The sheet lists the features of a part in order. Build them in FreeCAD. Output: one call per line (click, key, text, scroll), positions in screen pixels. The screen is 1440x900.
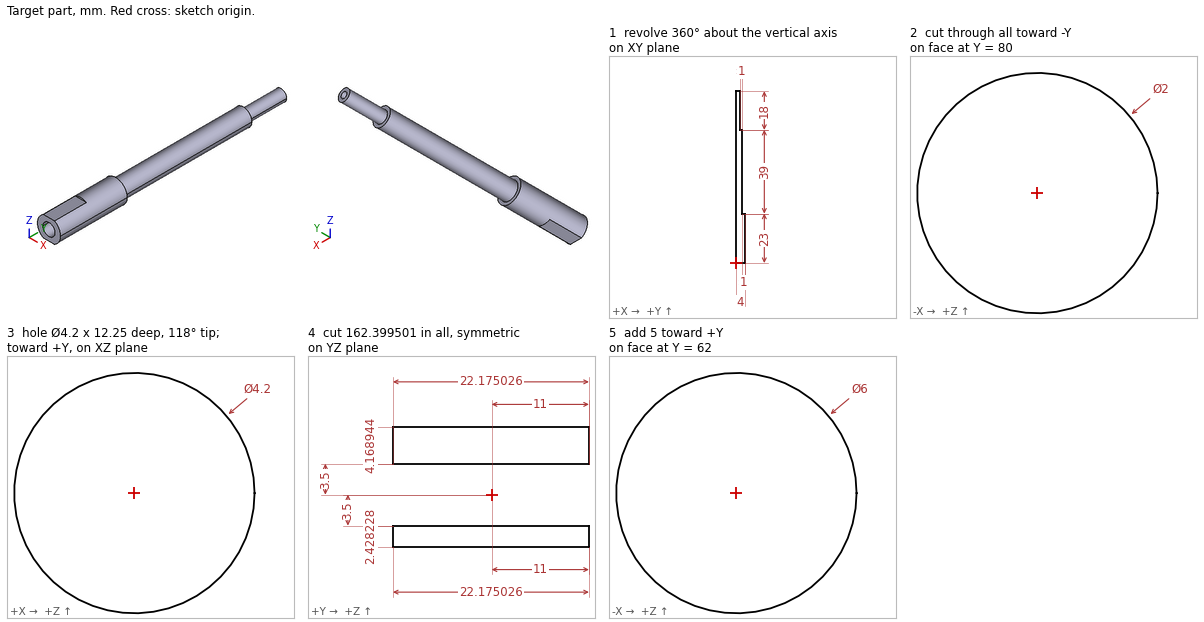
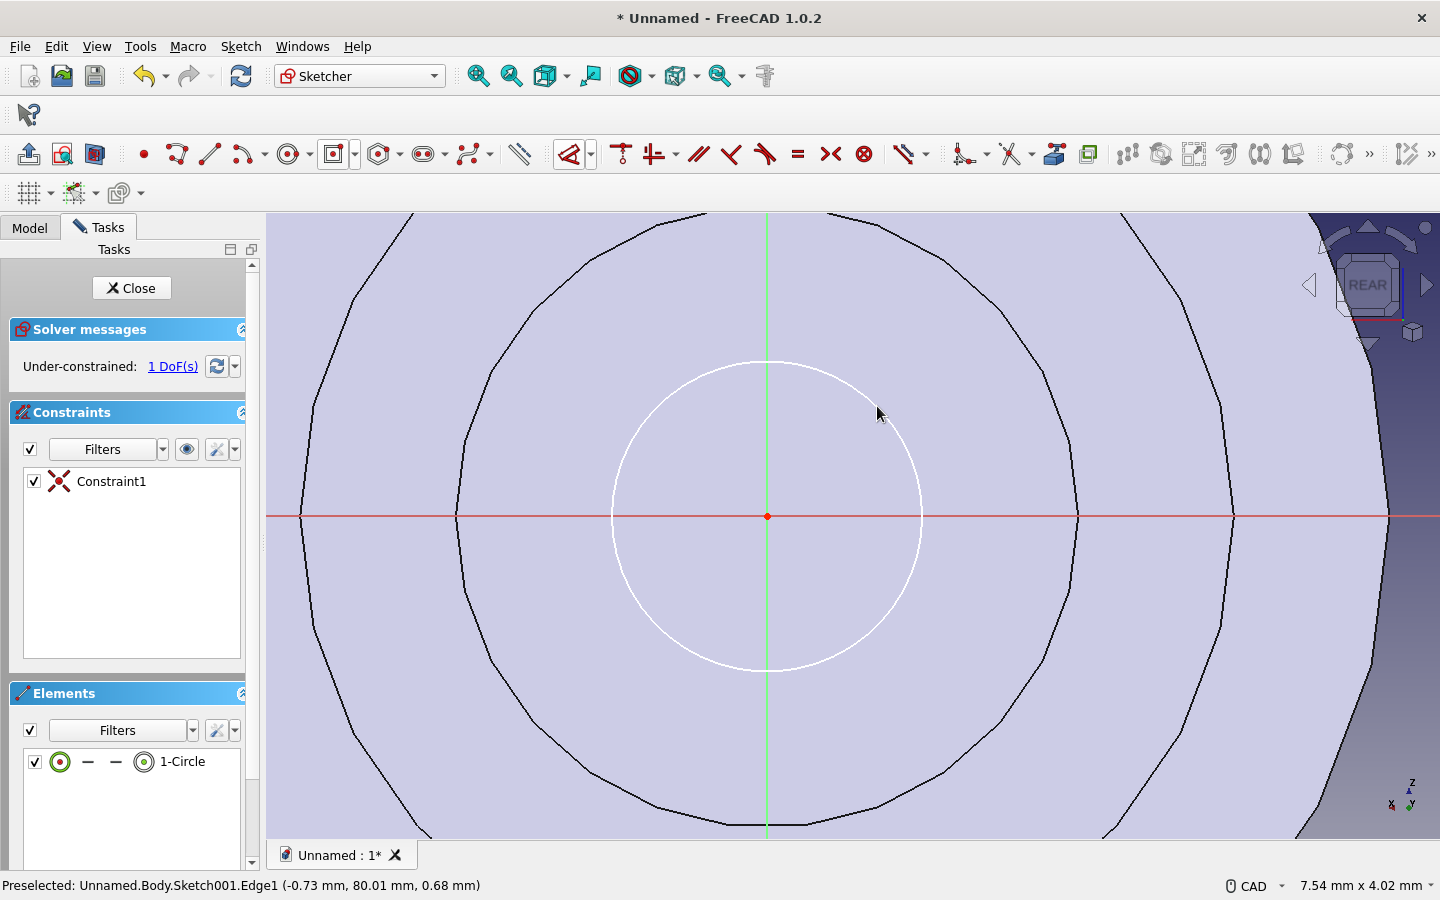
click(876, 406)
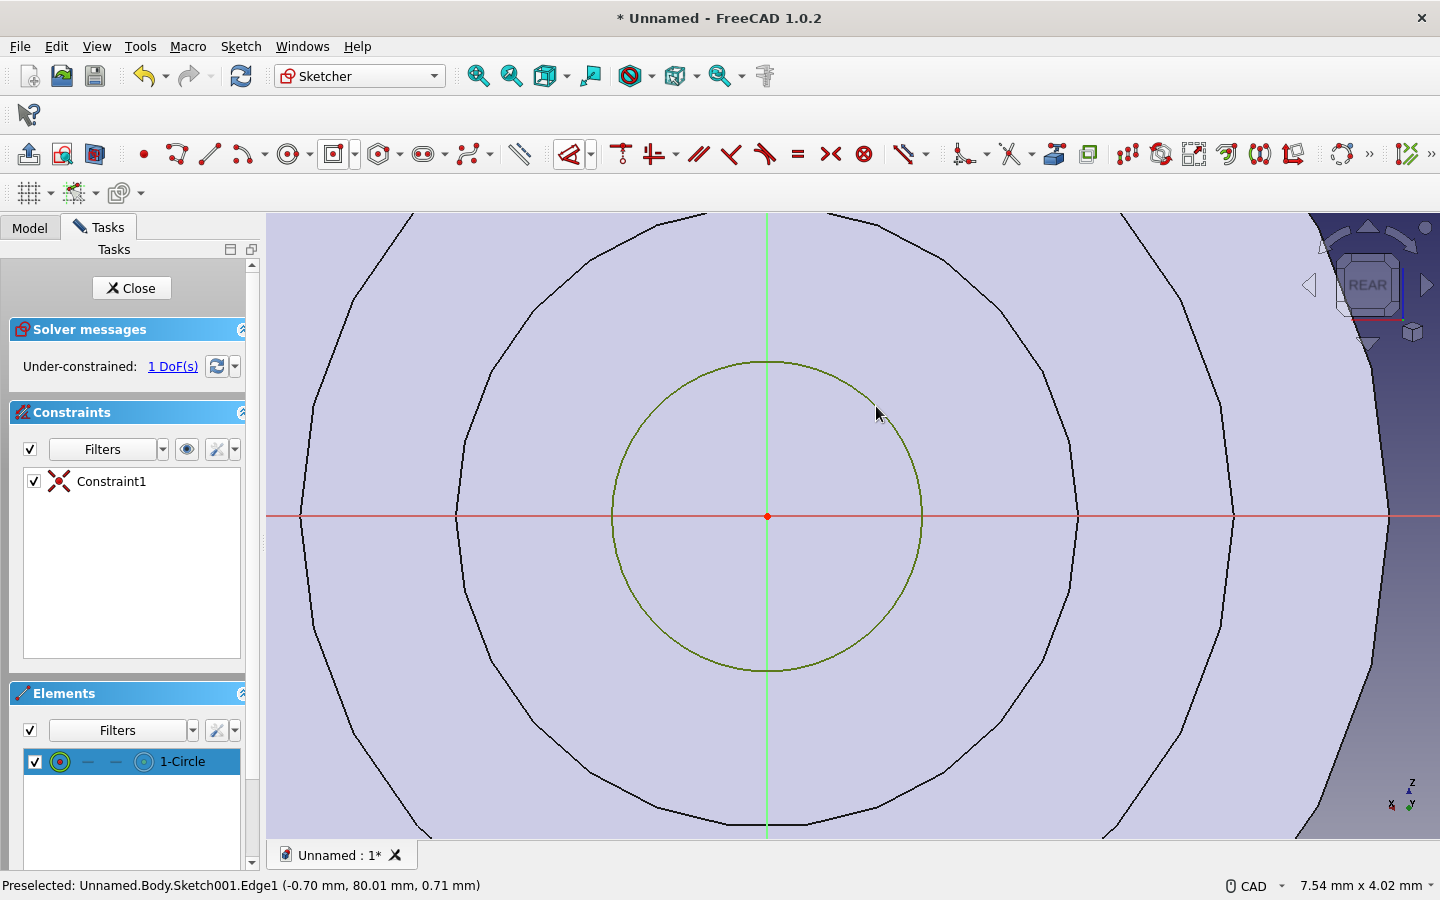
key(k)
key(o)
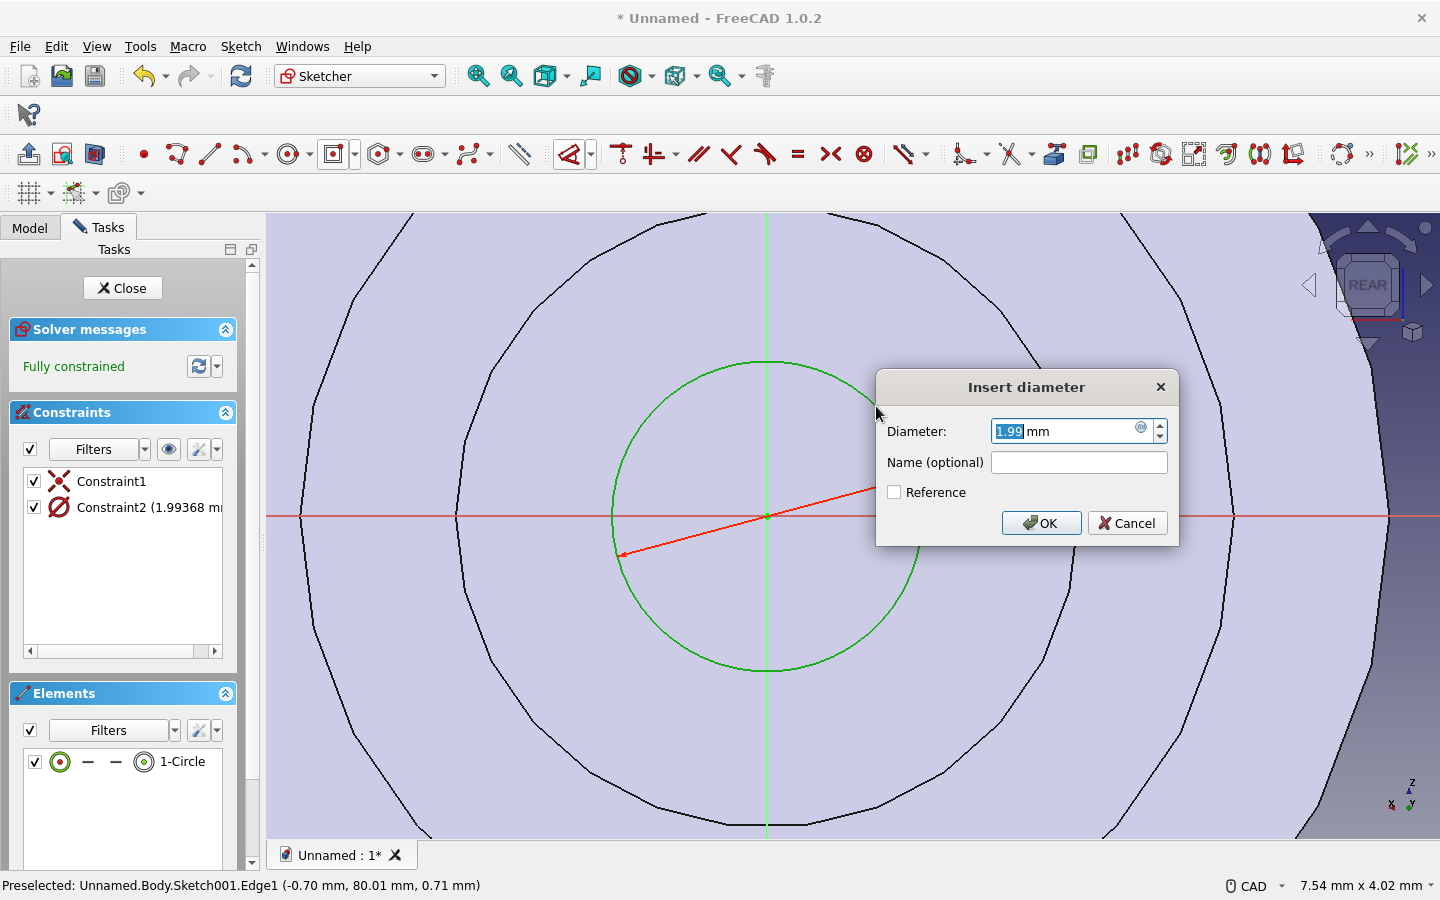
text(2)
key(Return)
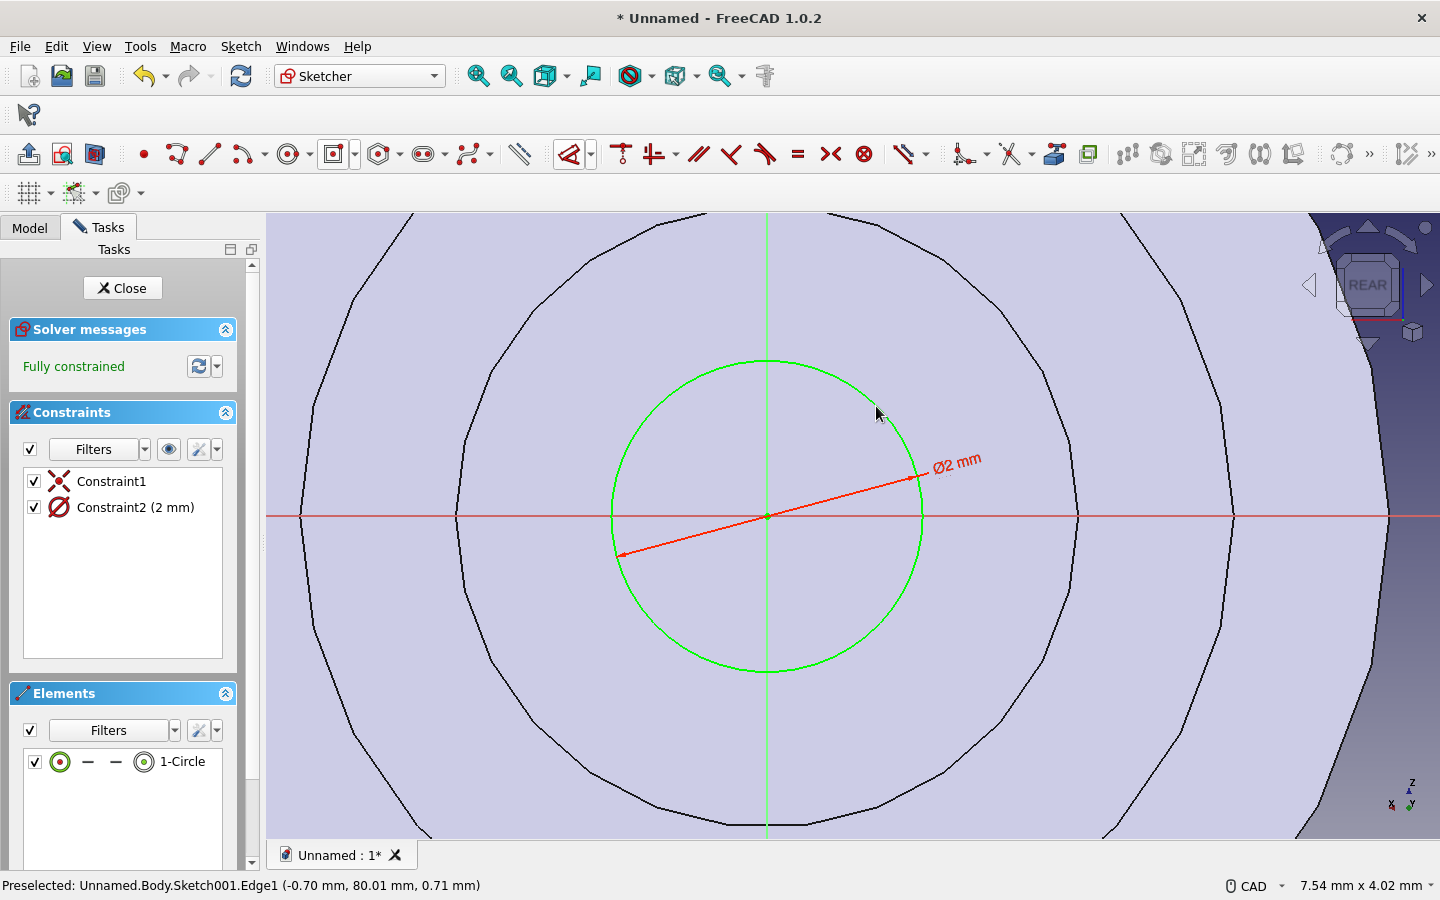
click(123, 288)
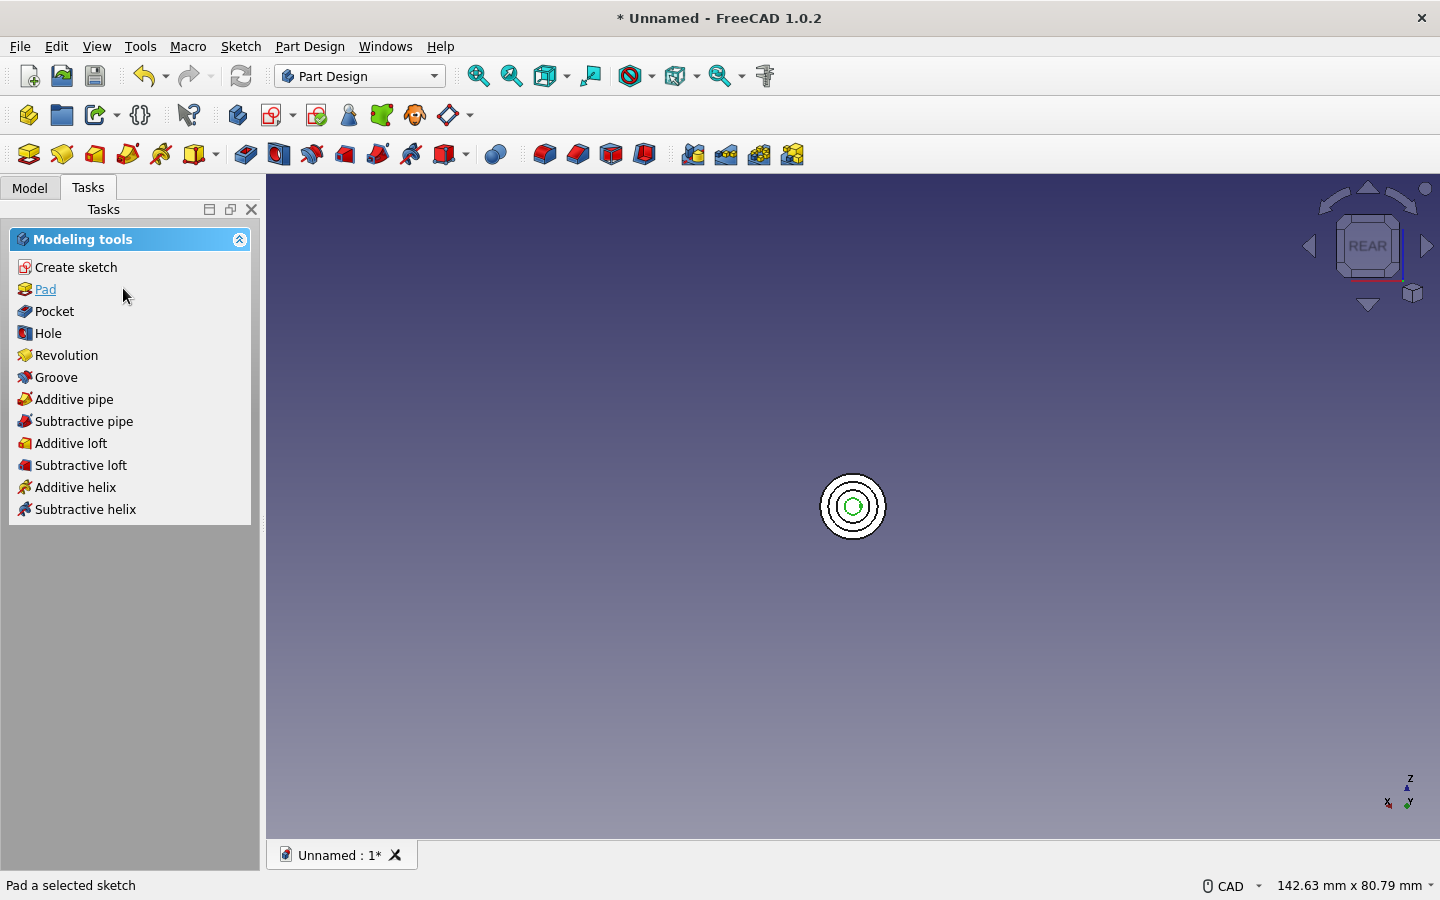
click(246, 154)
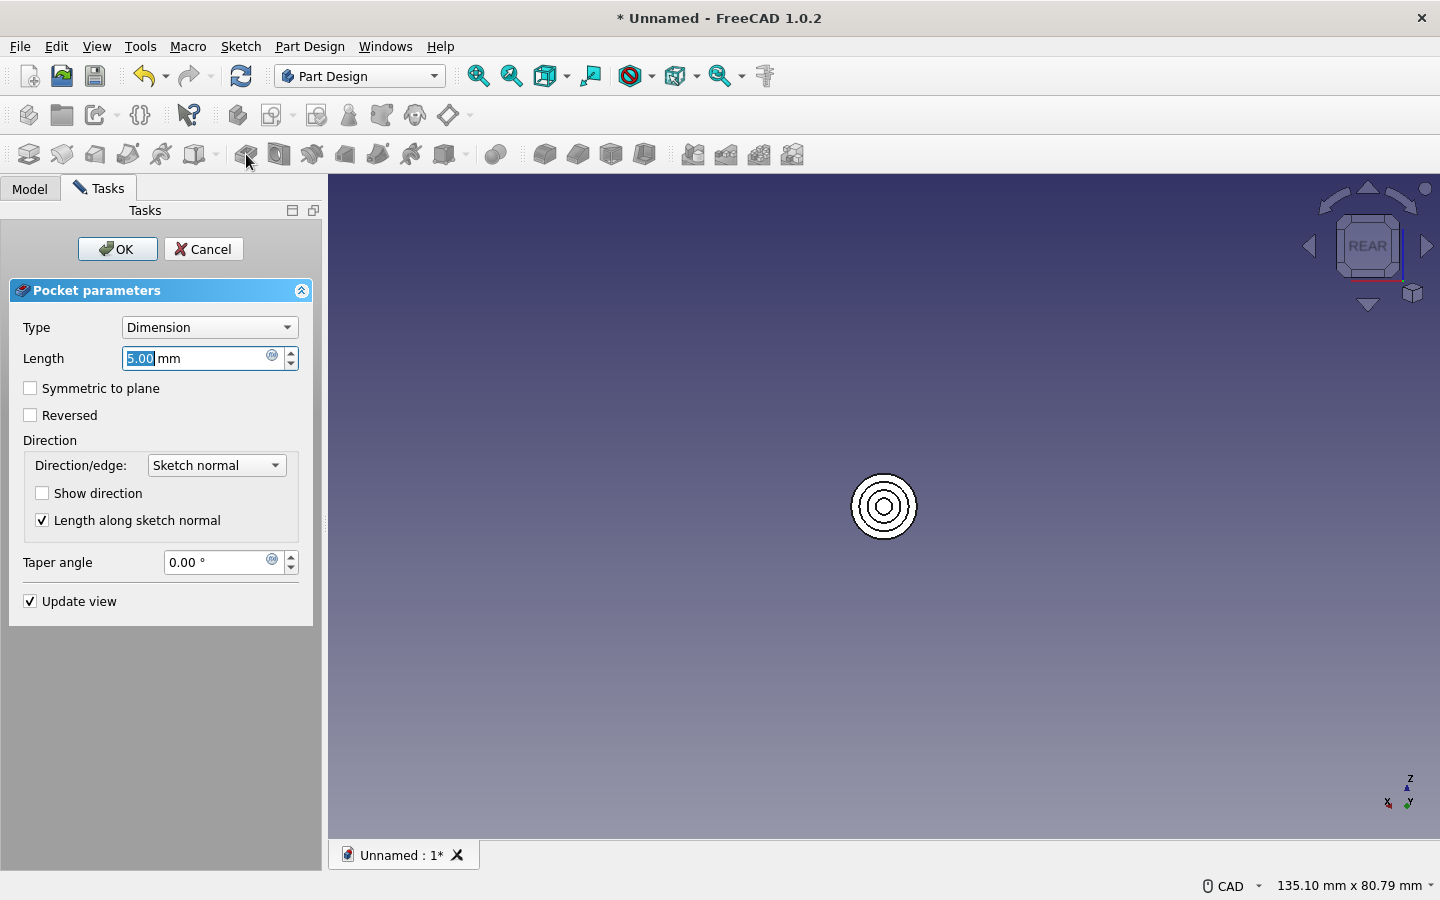
click(210, 328)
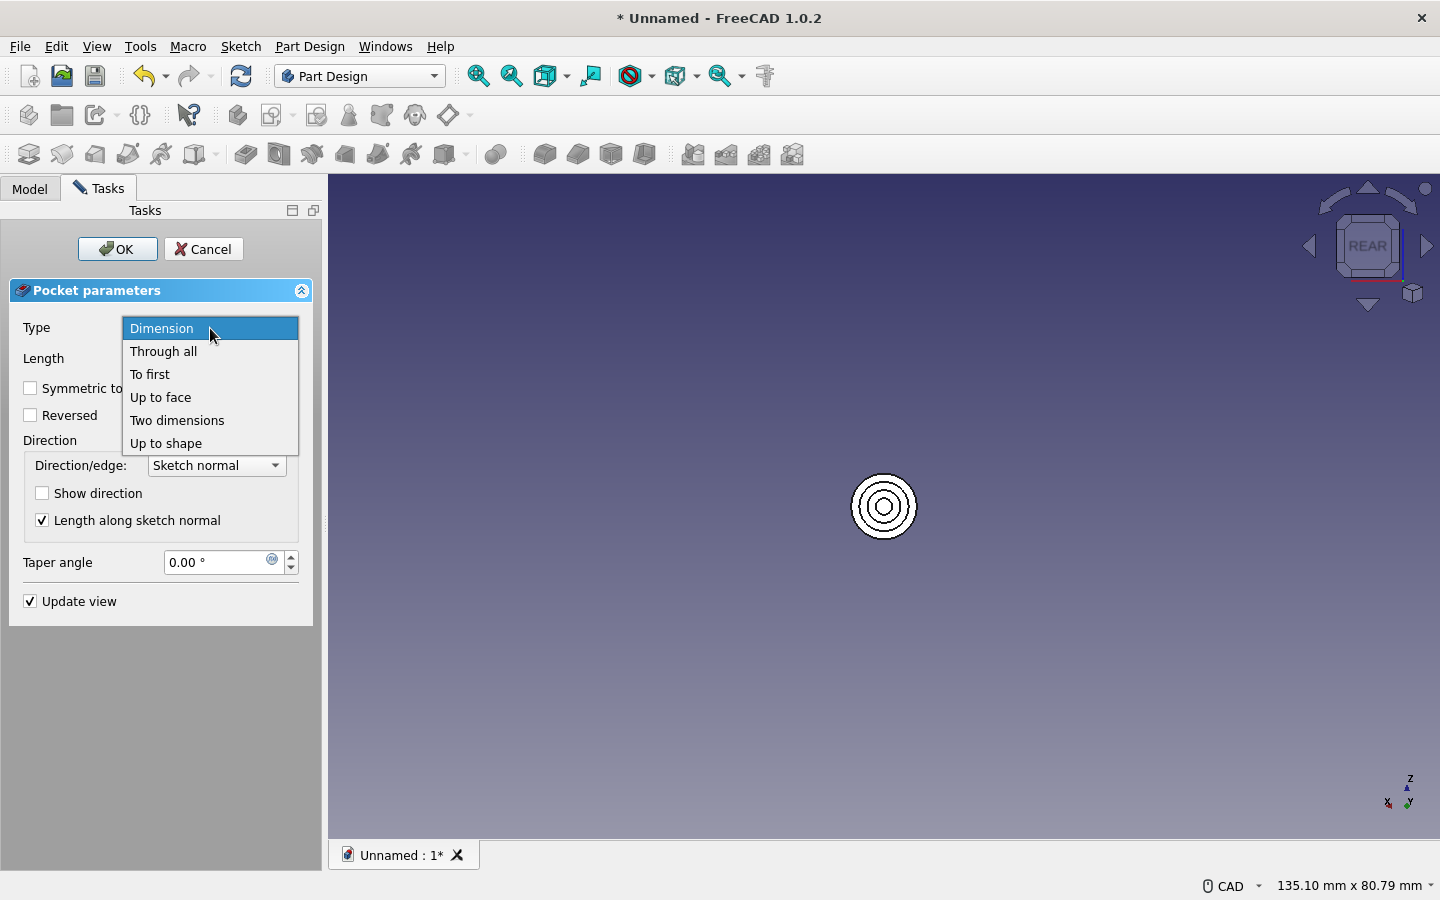
click(208, 352)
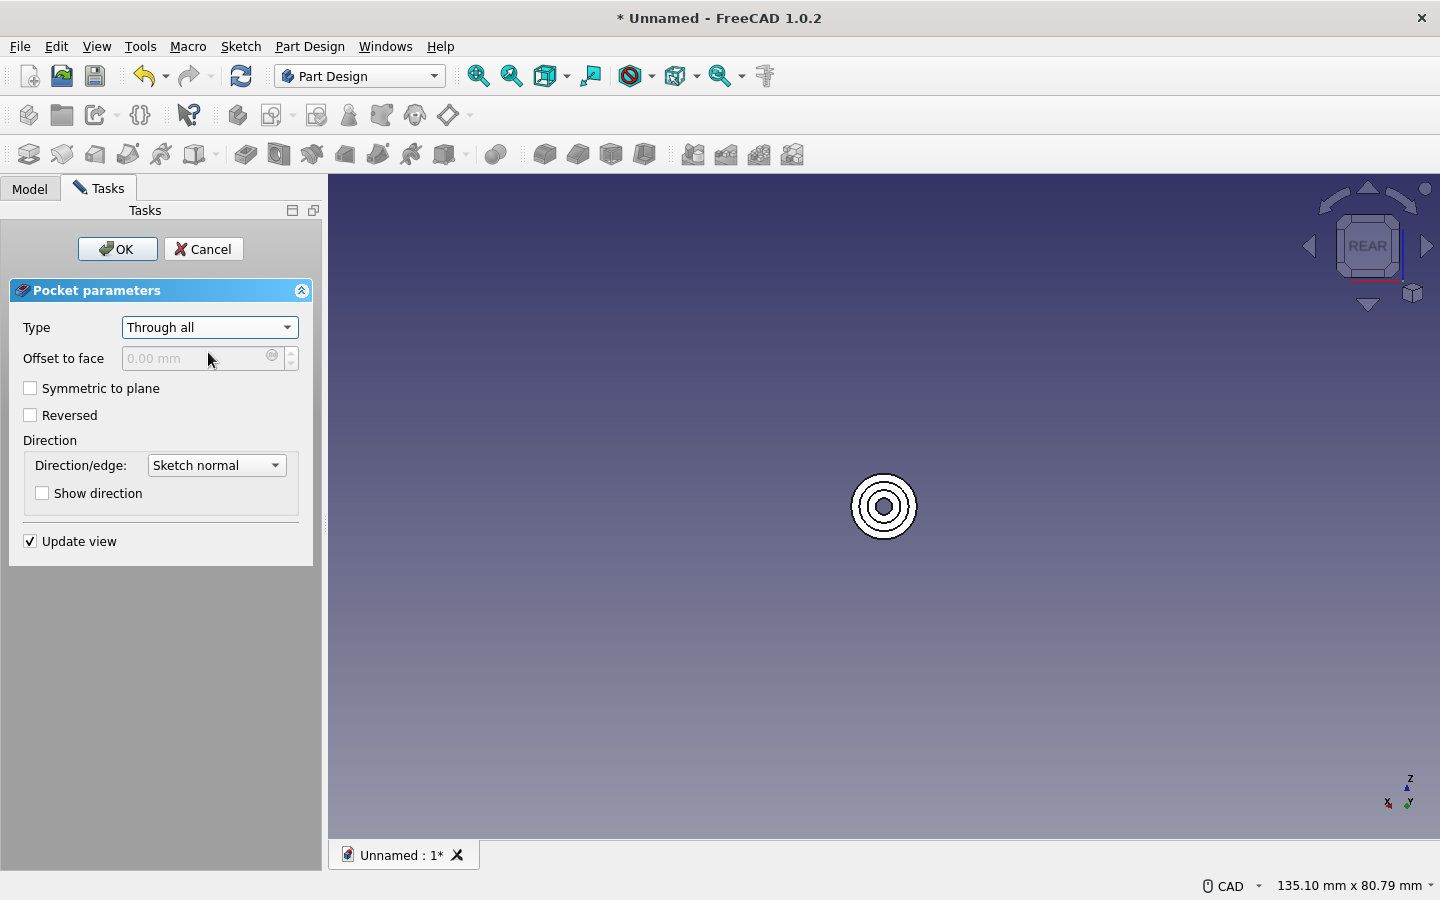
click(118, 249)